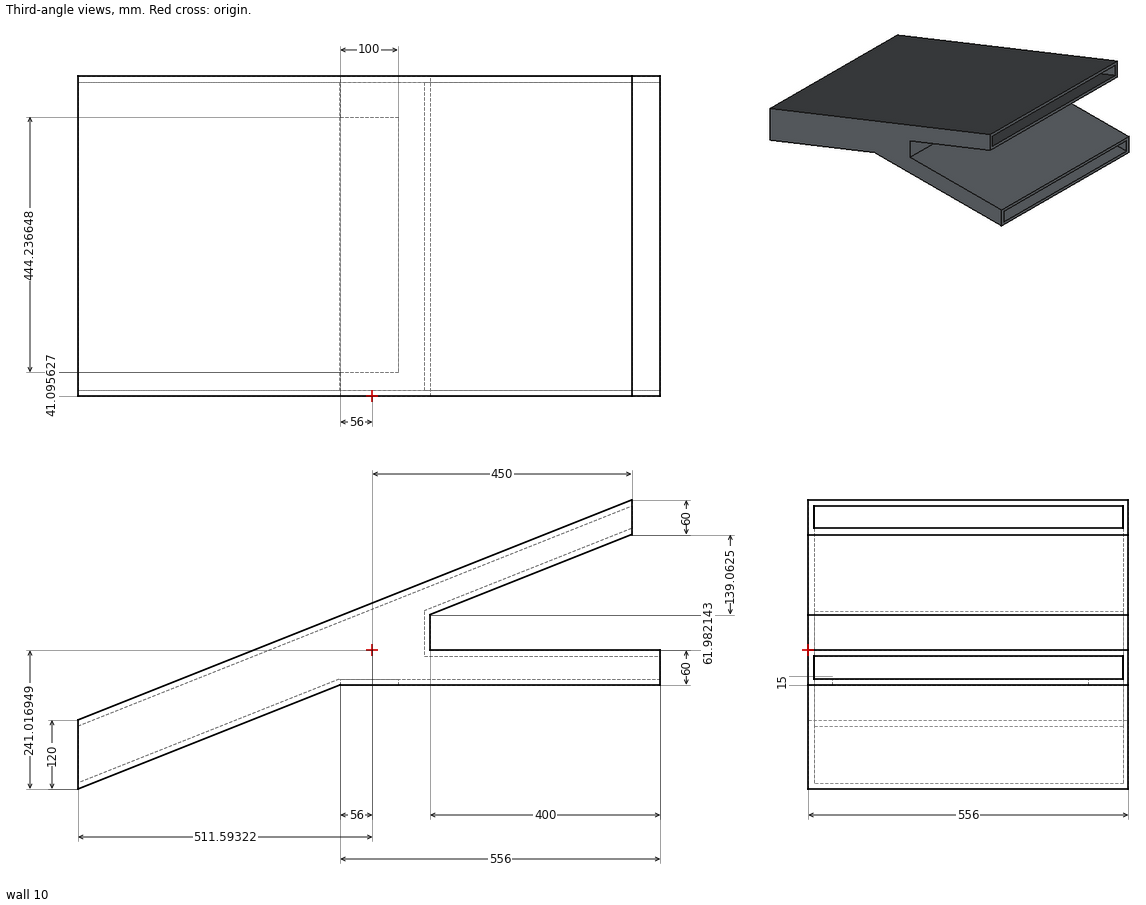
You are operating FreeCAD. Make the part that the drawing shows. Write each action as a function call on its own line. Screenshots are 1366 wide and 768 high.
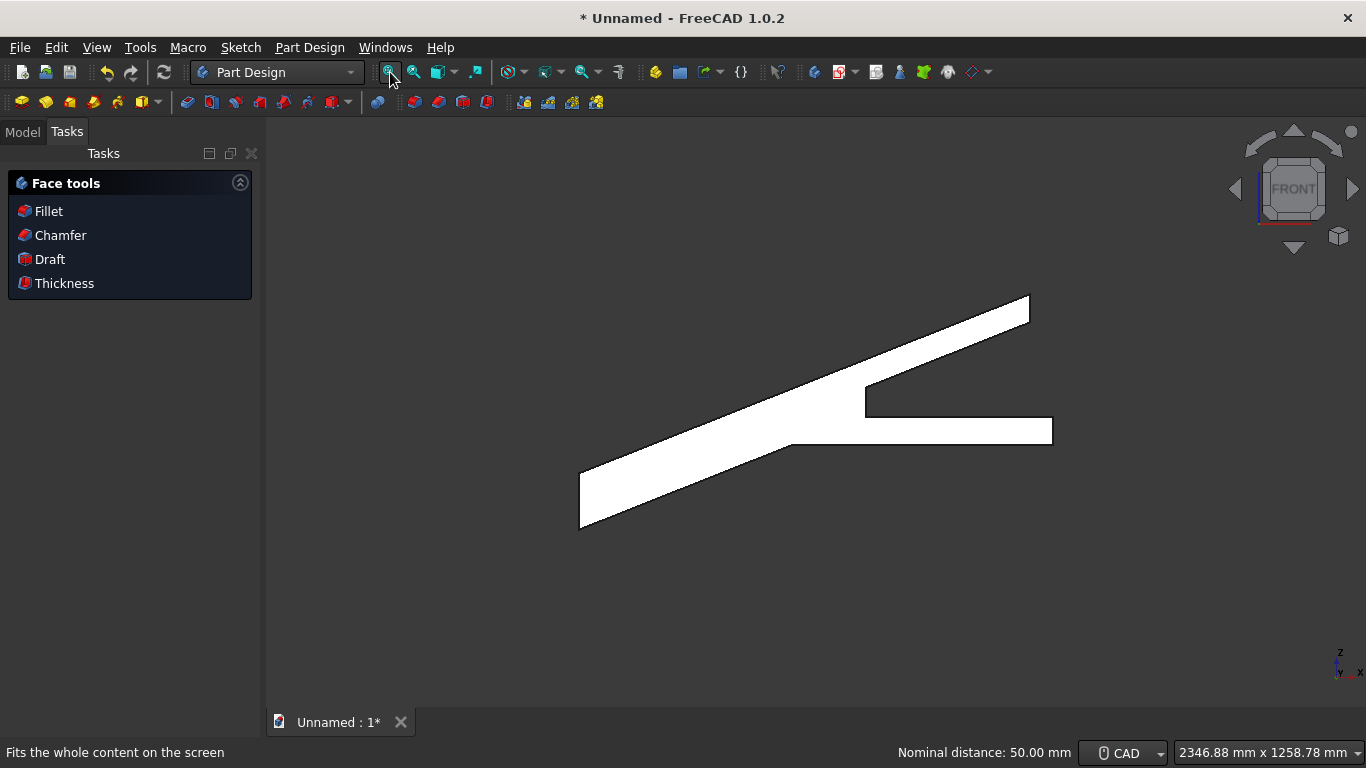
key(3)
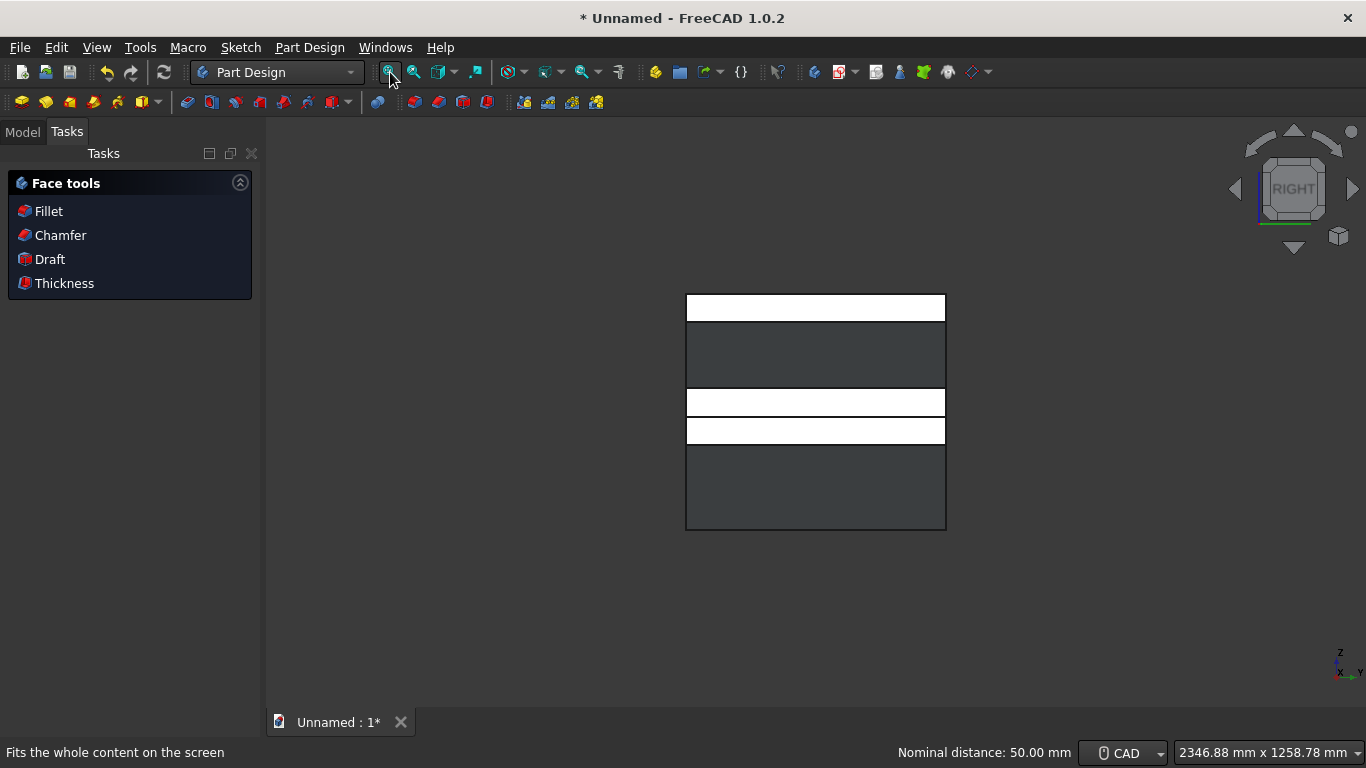
click(390, 72)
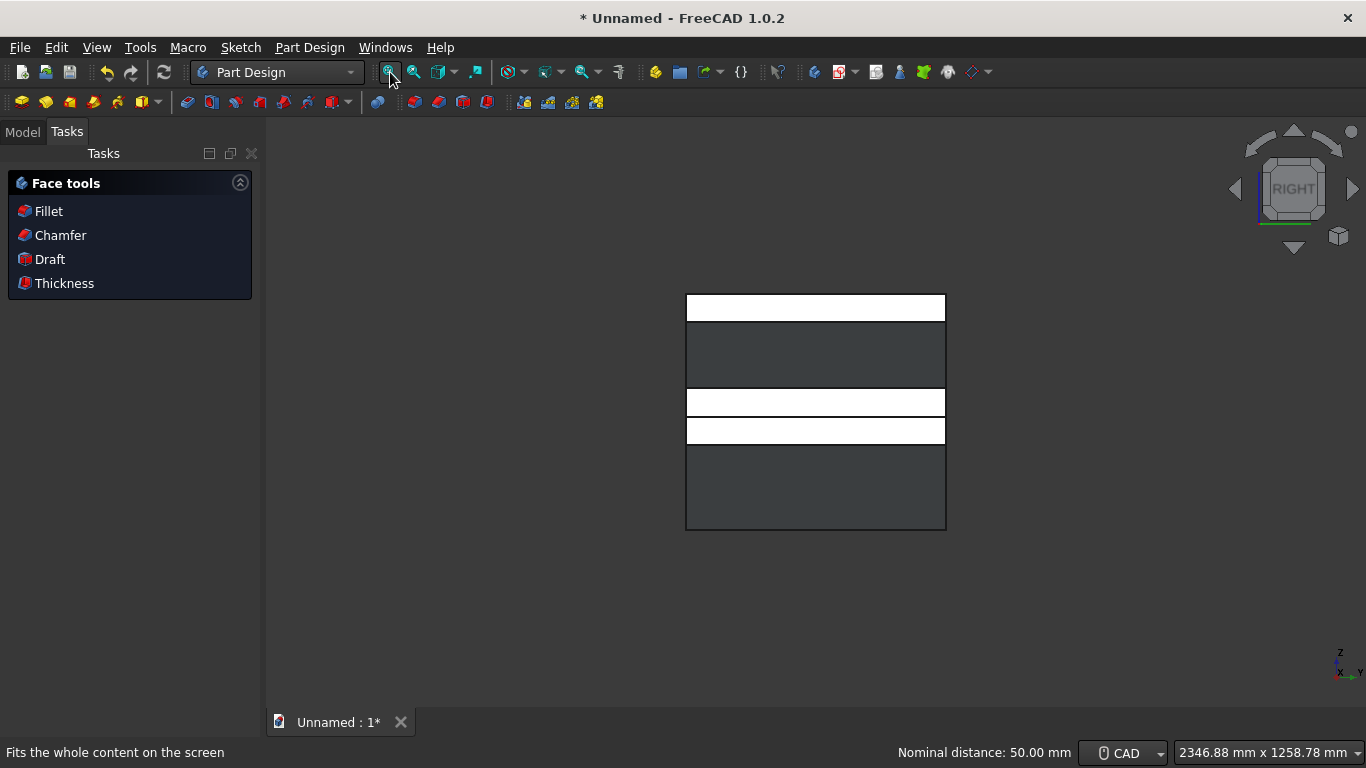
key(5)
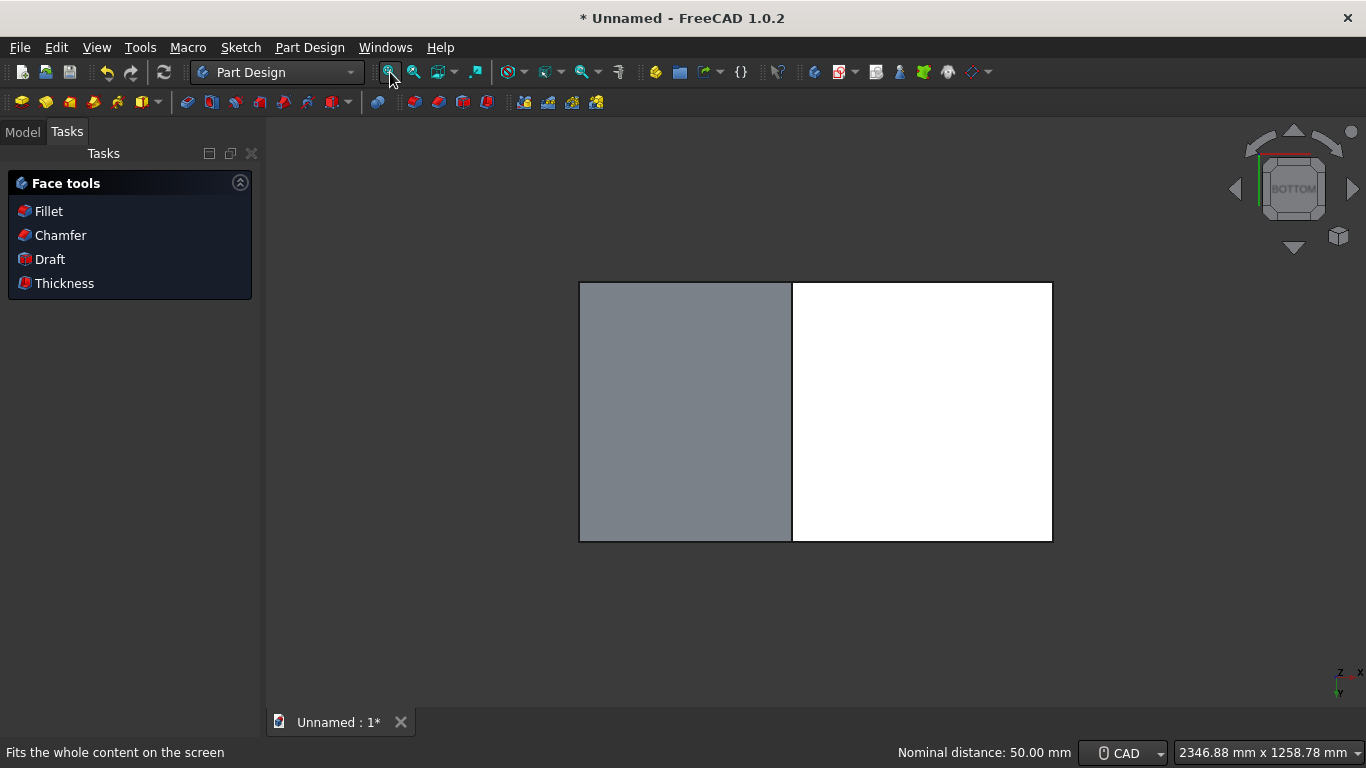
click(390, 72)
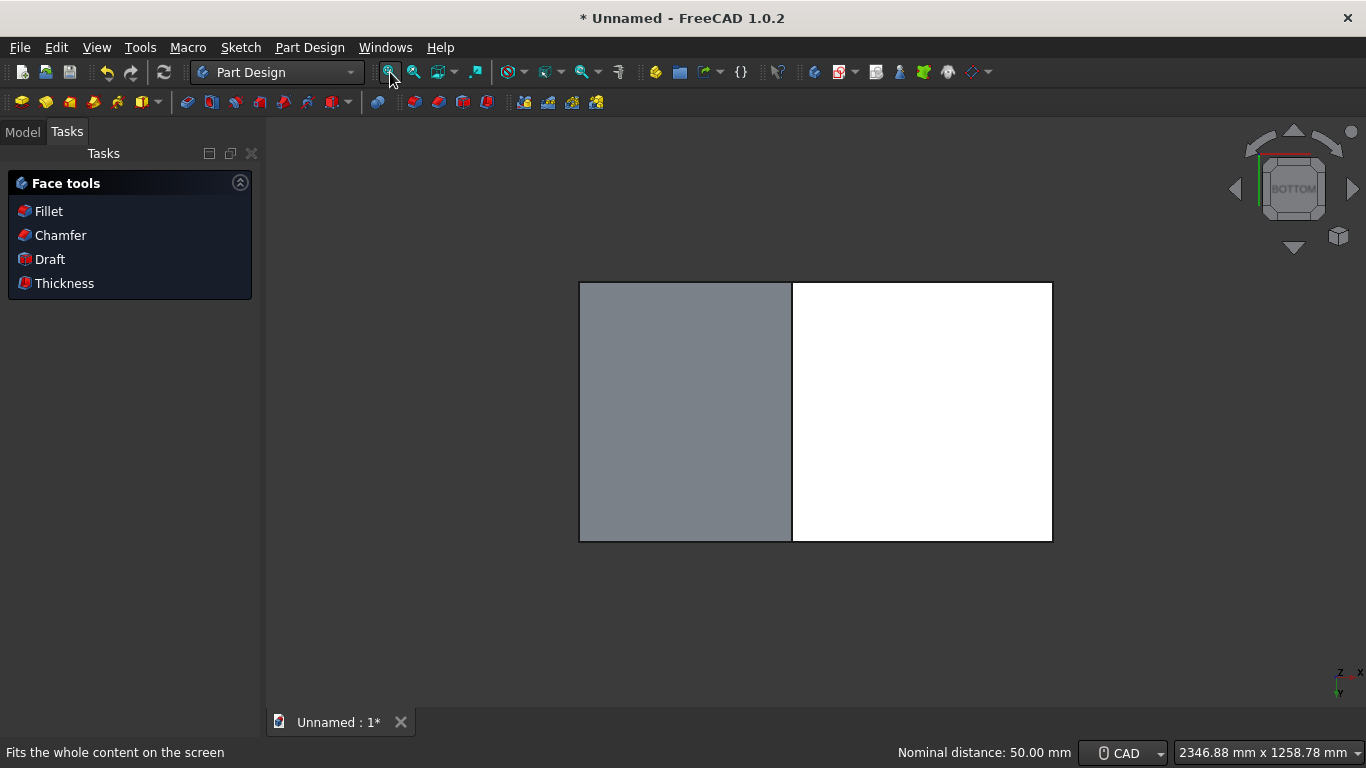
key(4)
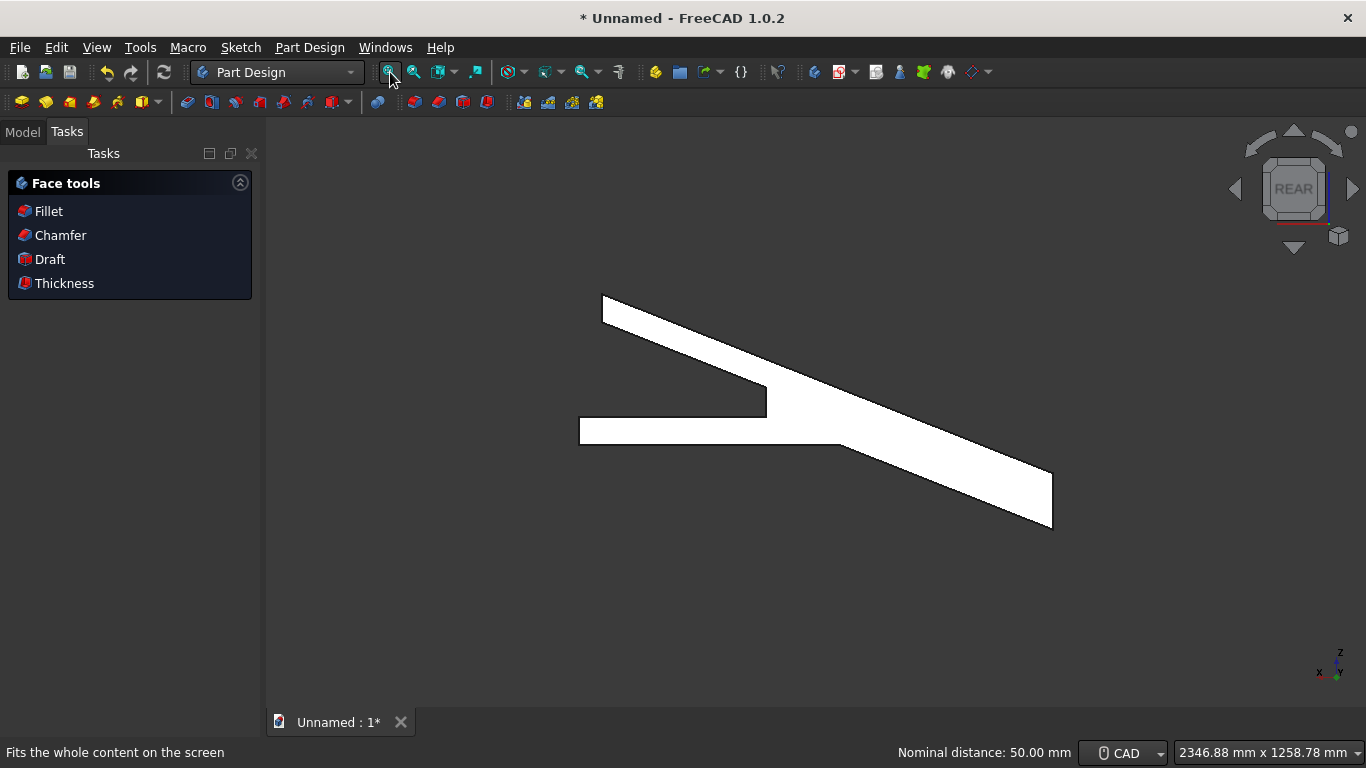
click(390, 72)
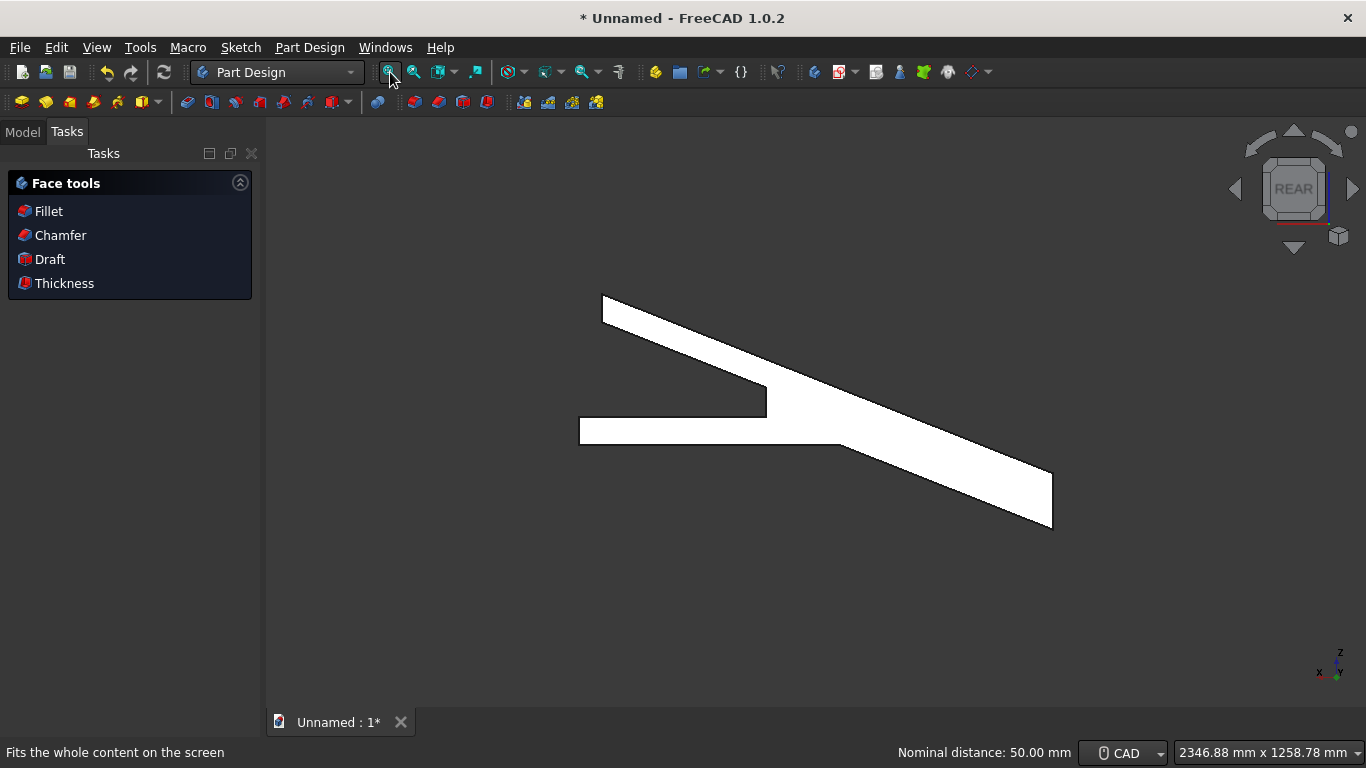
key(6)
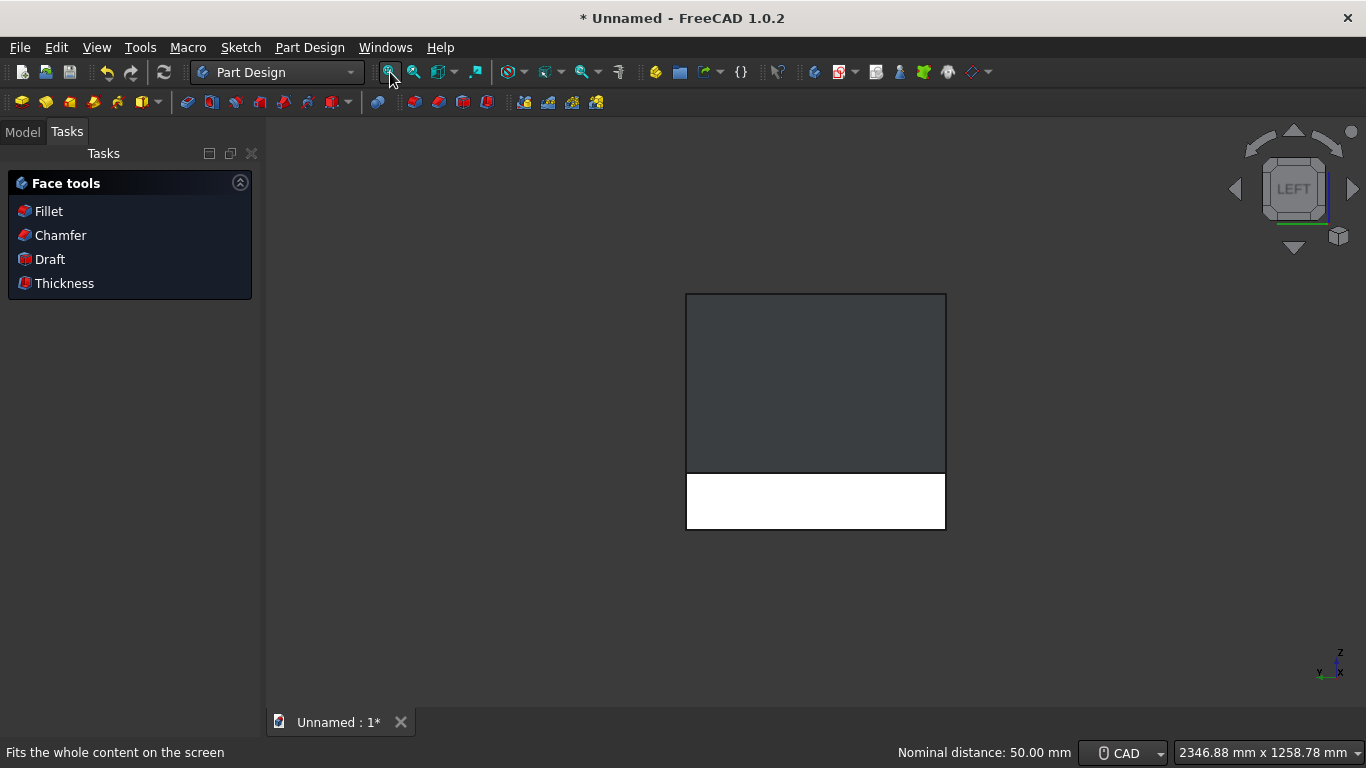
click(390, 72)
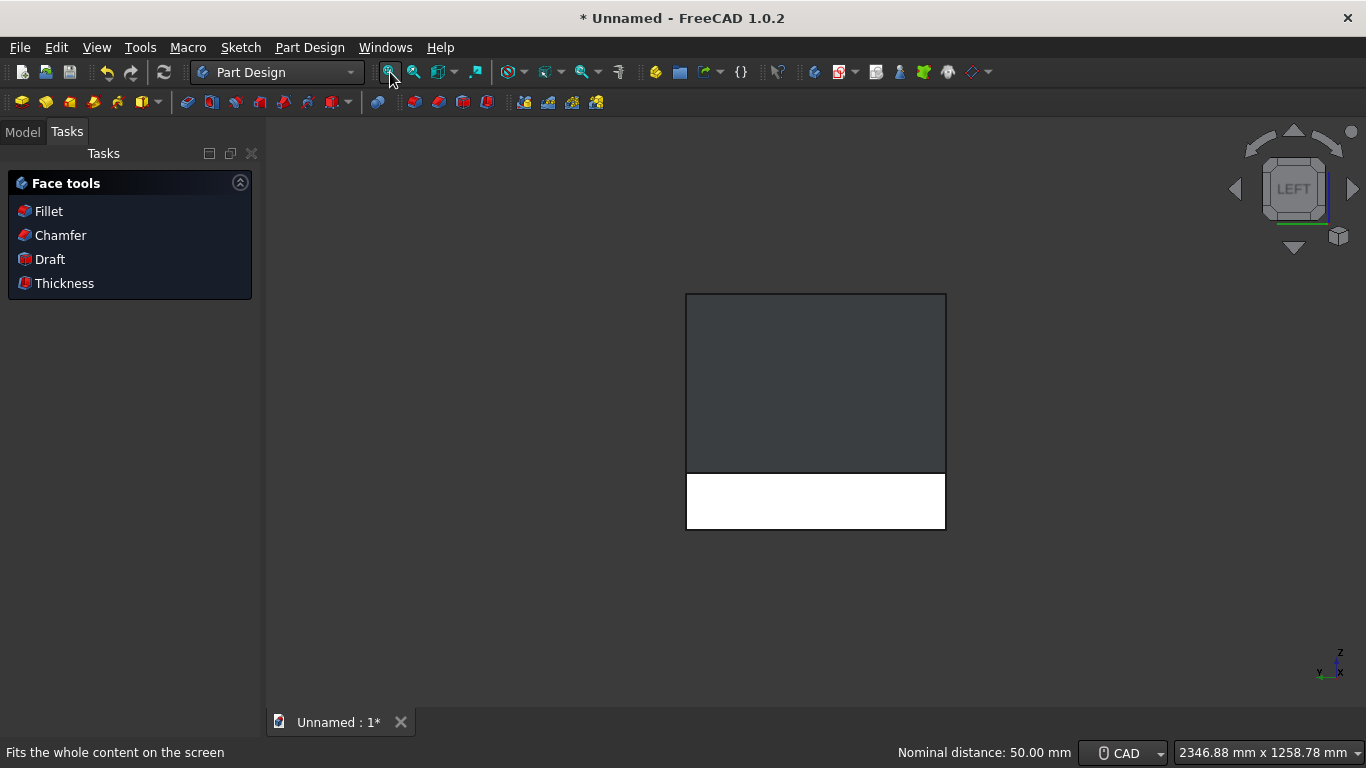
click(742, 501, ctrl)